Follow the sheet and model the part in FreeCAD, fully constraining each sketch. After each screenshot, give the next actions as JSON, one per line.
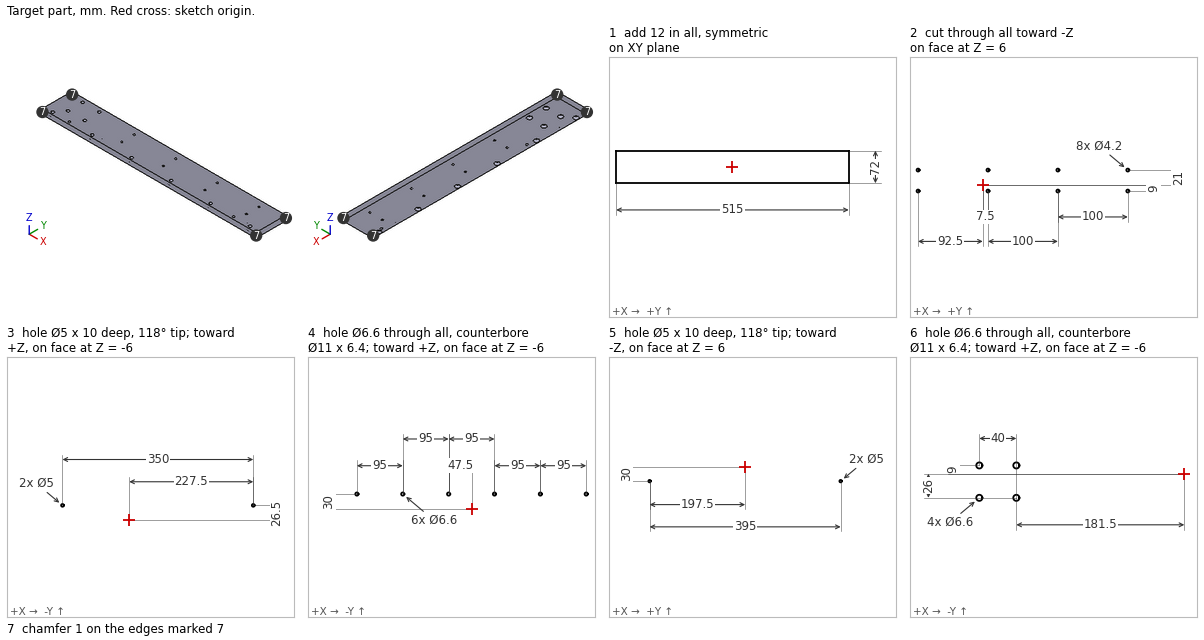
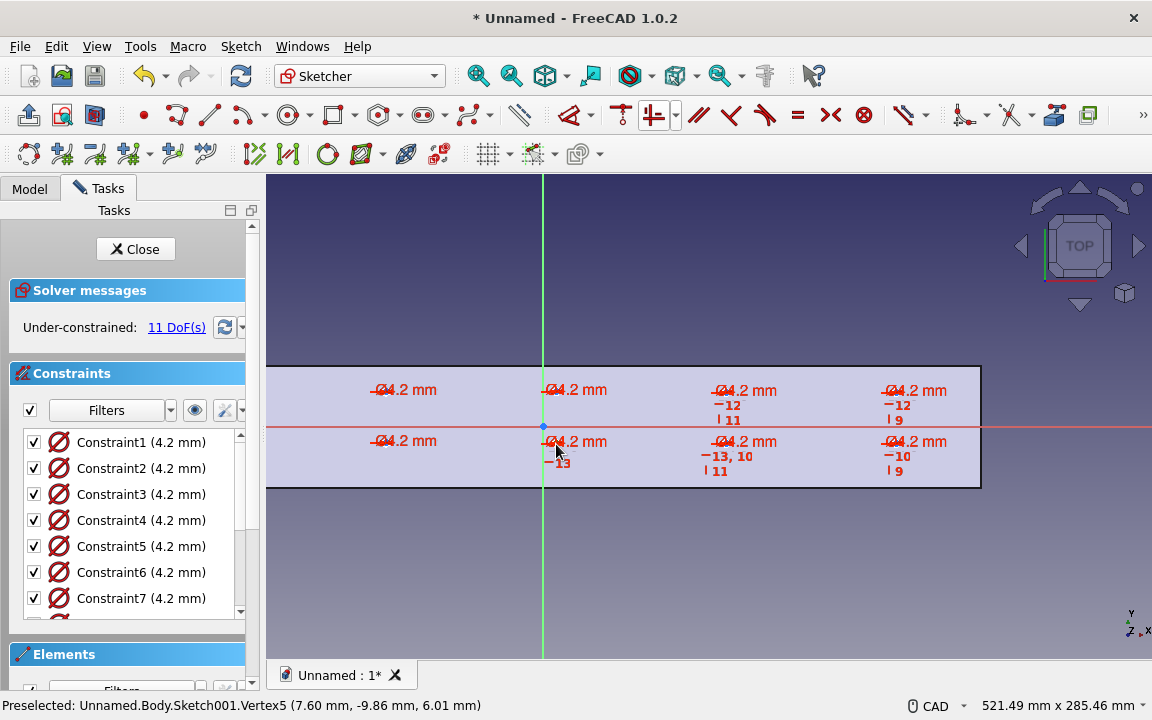
{"action": "left_click", "coordinate": [556, 392]}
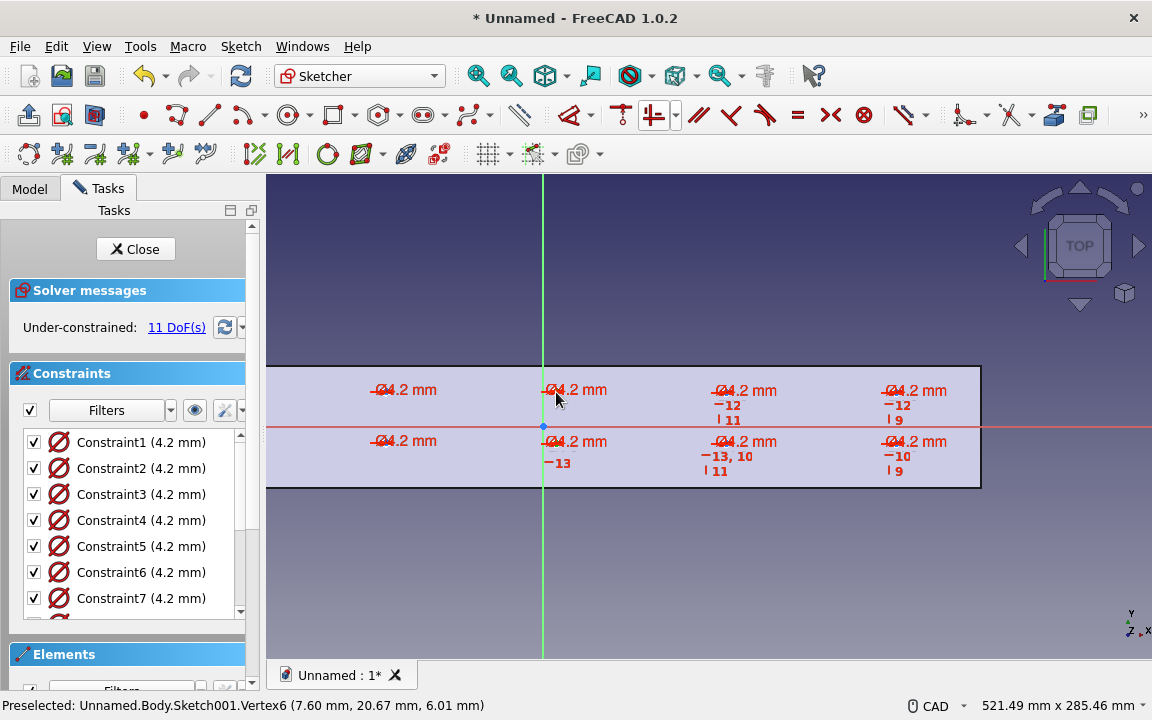
{"action": "left_click", "coordinate": [676, 116]}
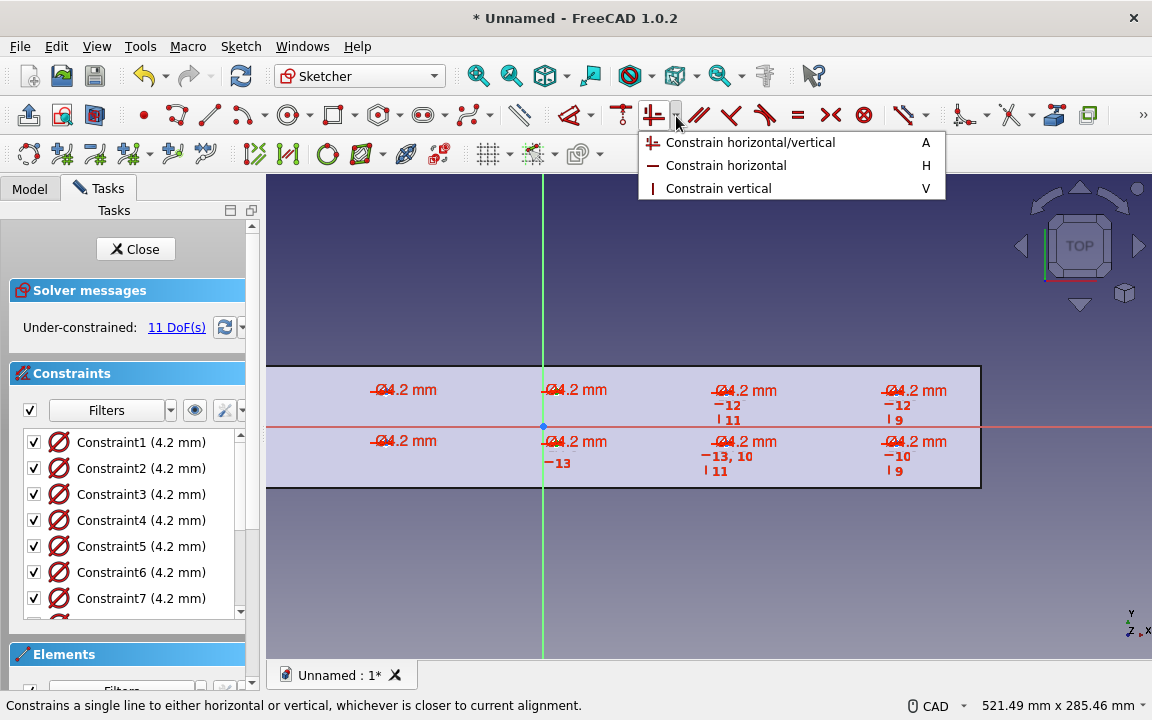
{"action": "left_click", "coordinate": [792, 188]}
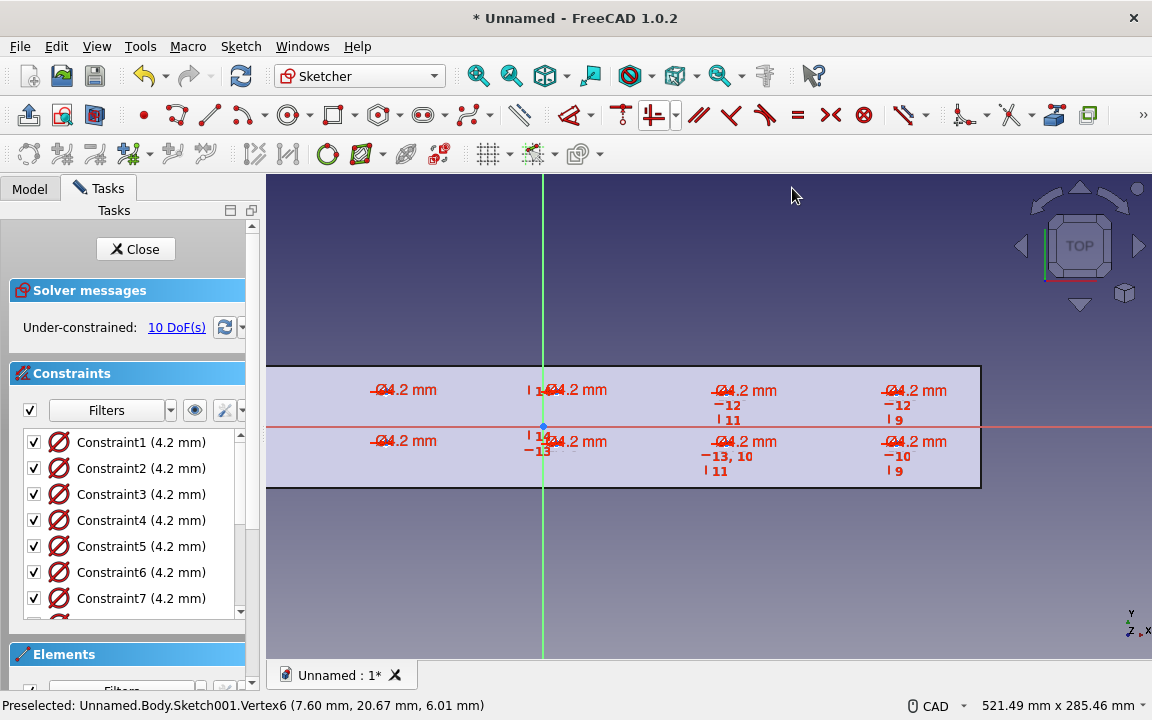
{"action": "left_click", "coordinate": [726, 393]}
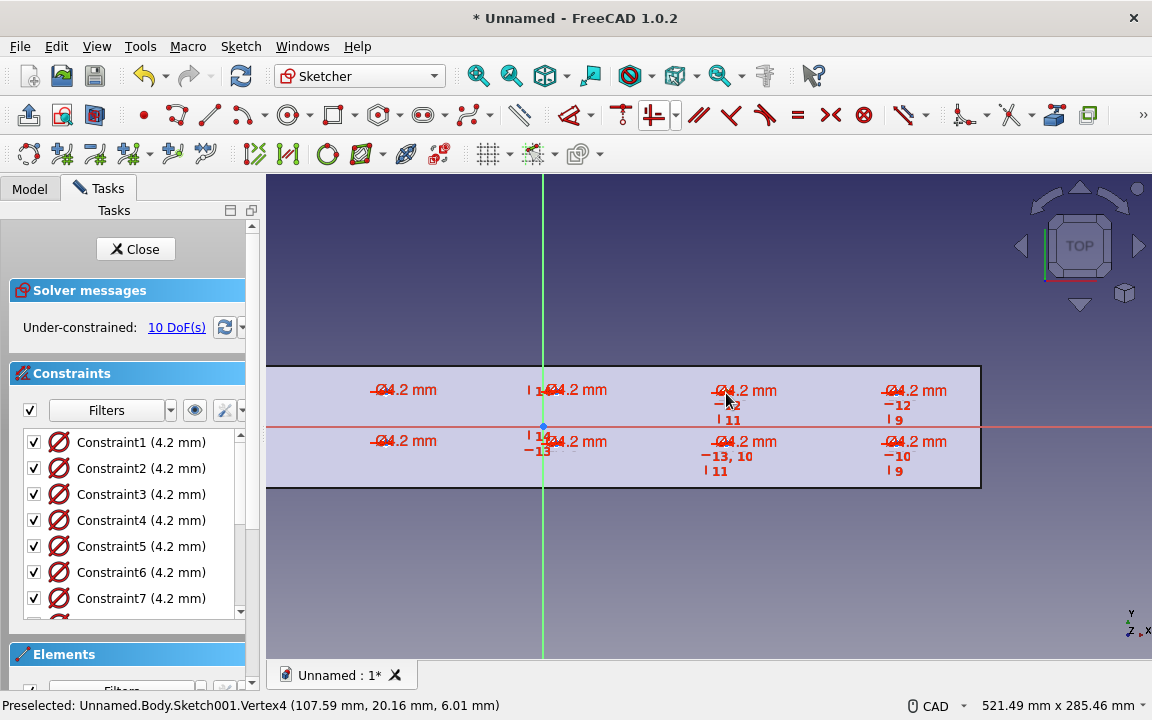
{"action": "left_click", "coordinate": [556, 392]}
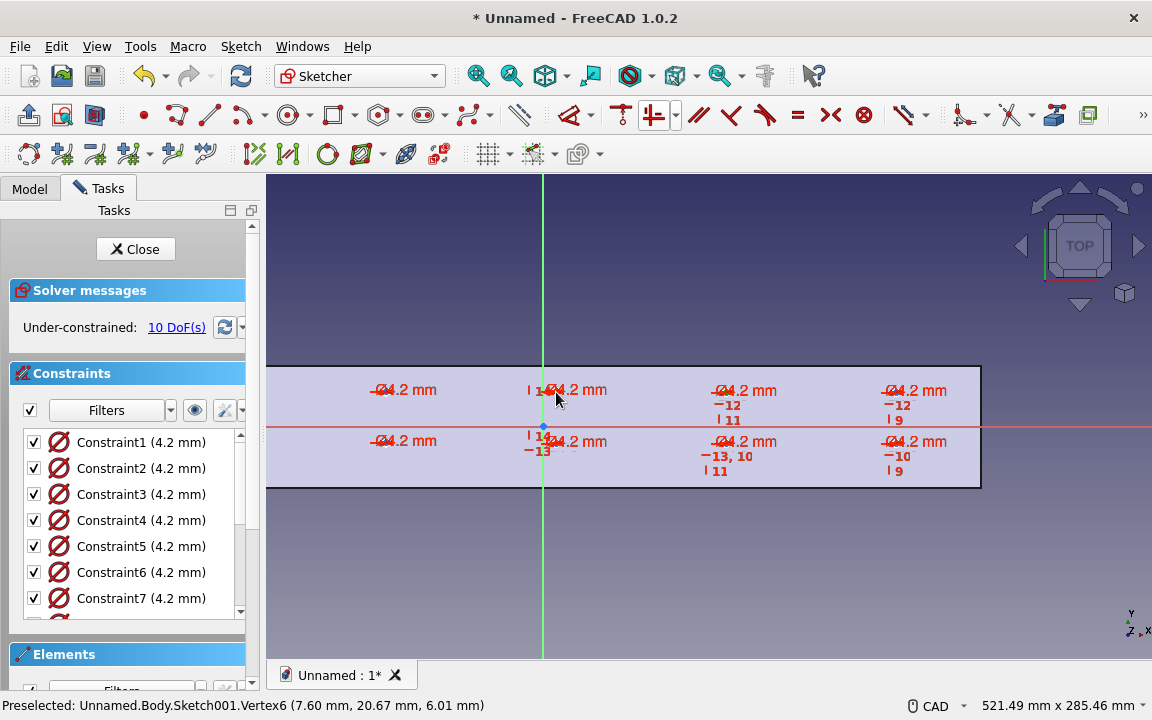
{"action": "key", "text": "h"}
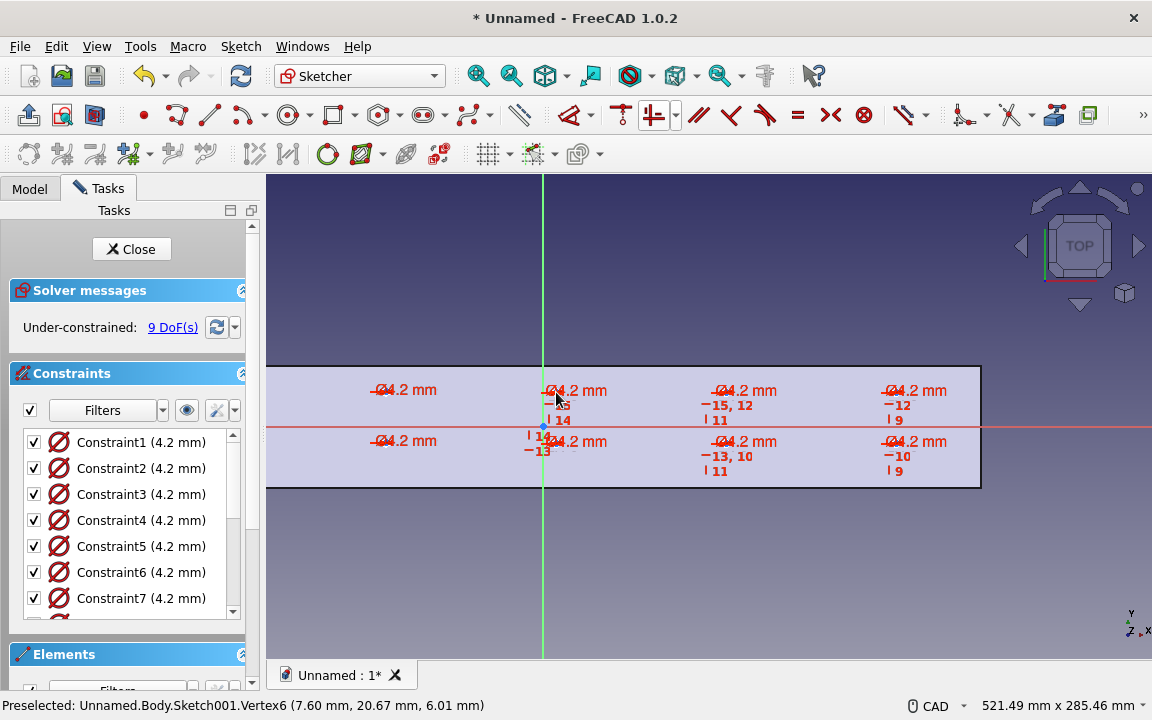
{"action": "left_click", "coordinate": [556, 444]}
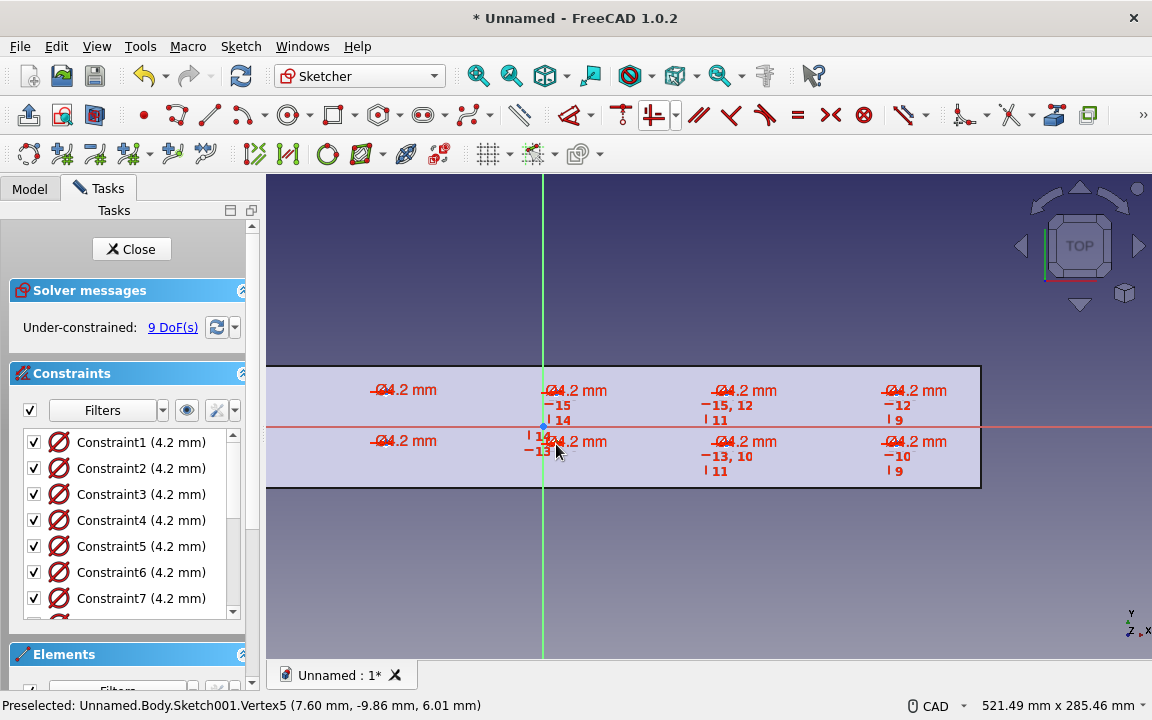
{"action": "left_click", "coordinate": [386, 443]}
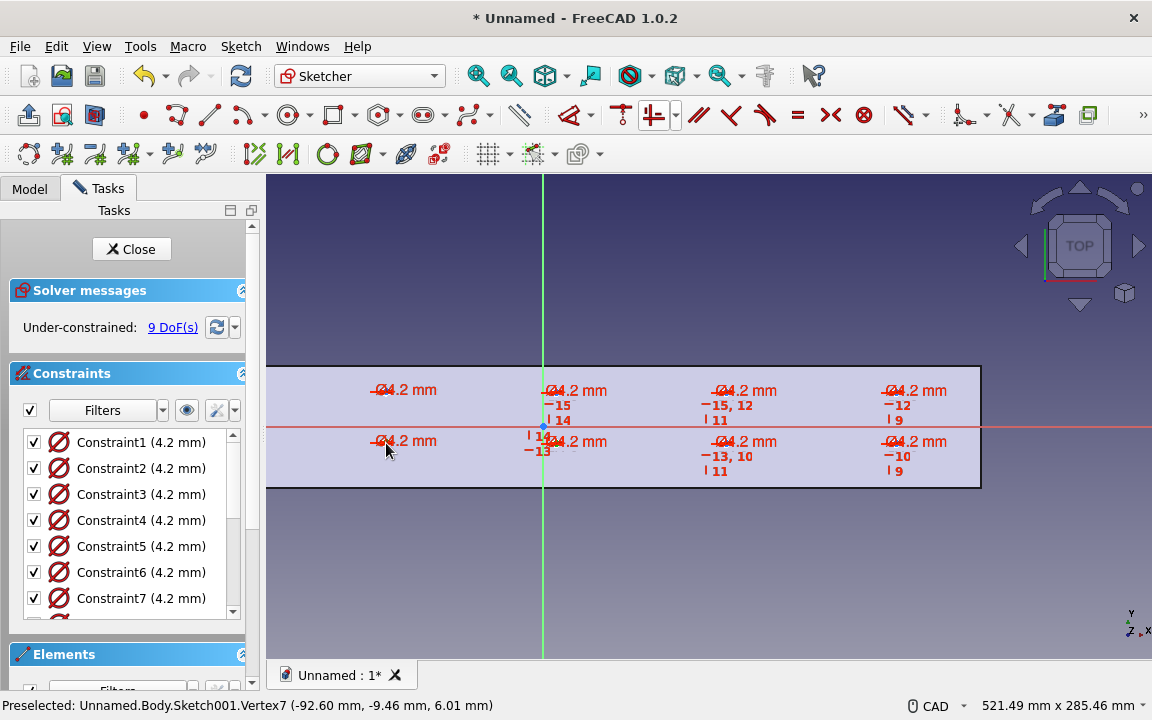
{"action": "left_click", "coordinate": [676, 116]}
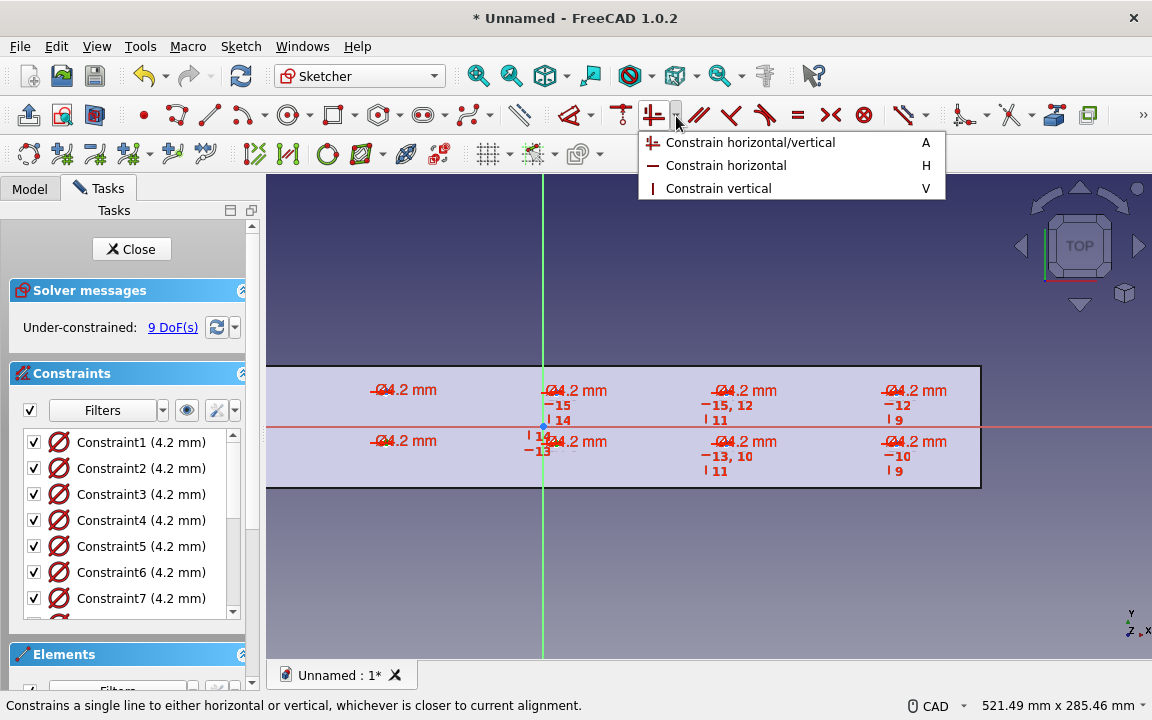
{"action": "left_click", "coordinate": [792, 166]}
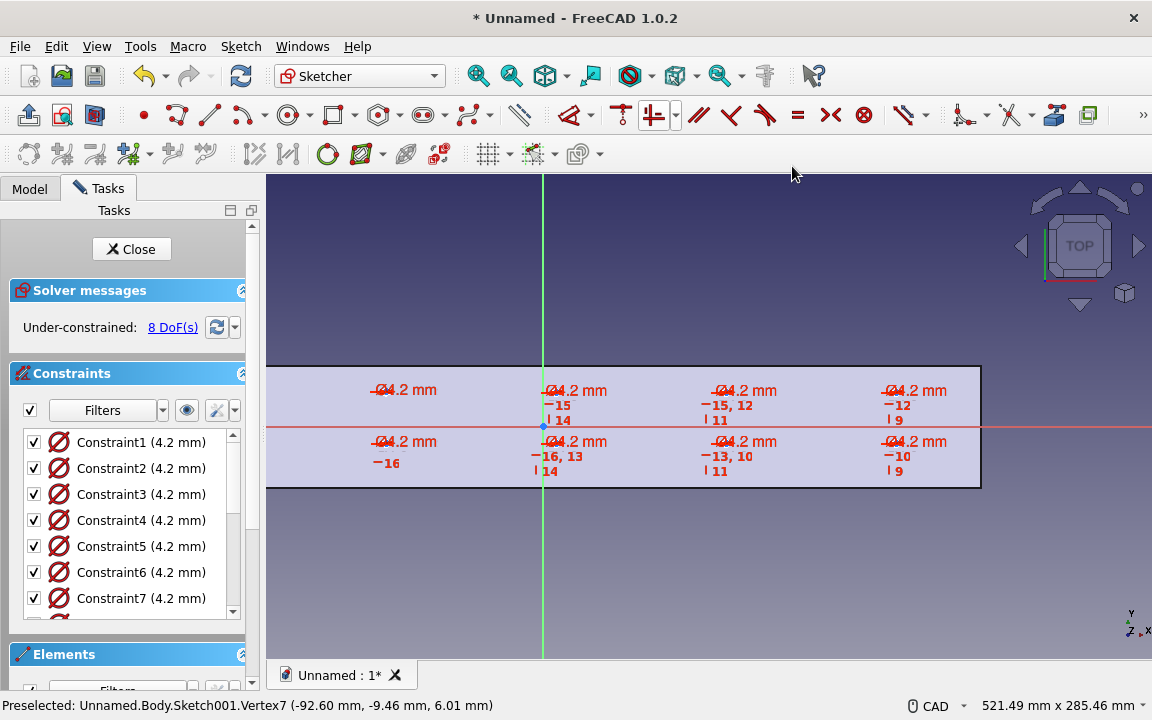
{"action": "left_click", "coordinate": [386, 444]}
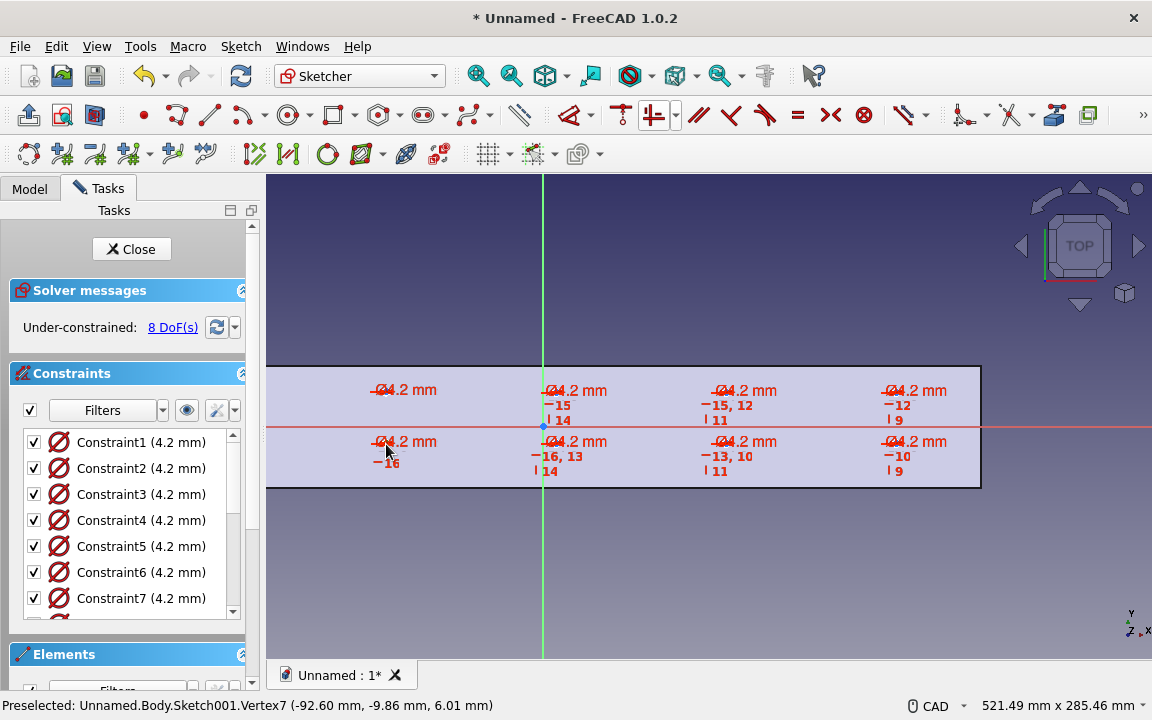
{"action": "left_click", "coordinate": [386, 392]}